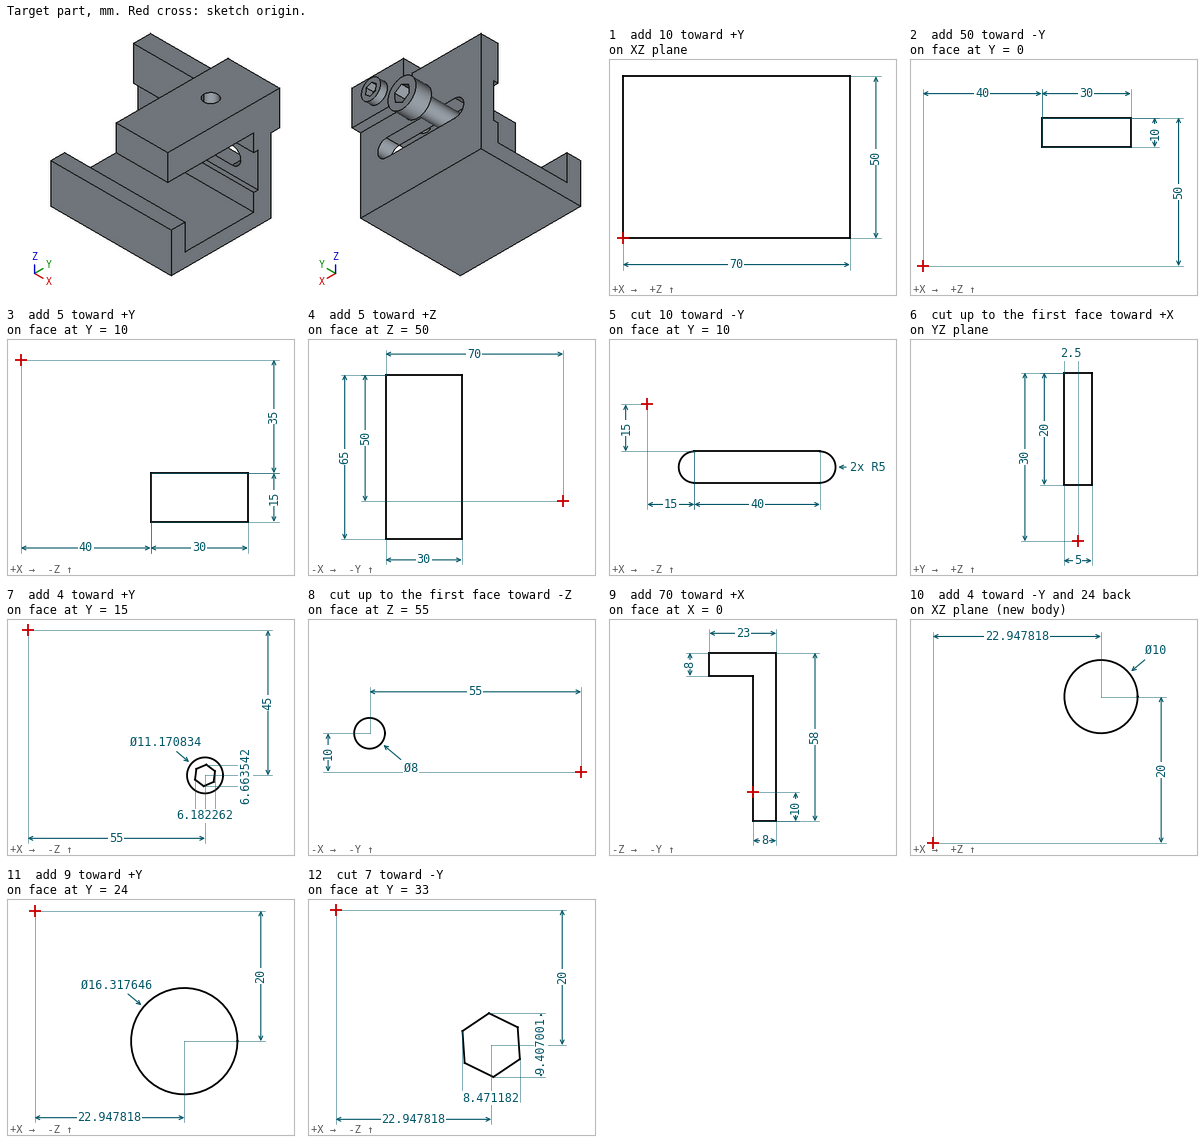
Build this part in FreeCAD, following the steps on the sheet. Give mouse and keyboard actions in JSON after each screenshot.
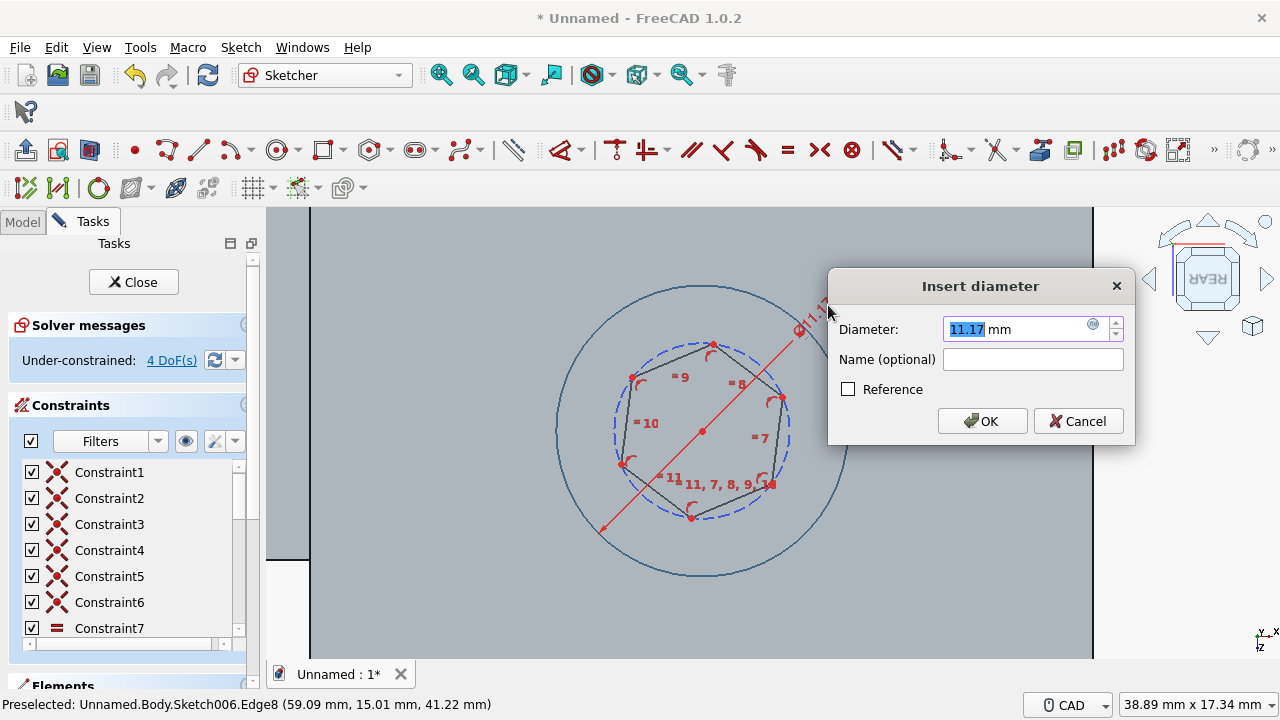
{"action": "type", "text": "11.170834"}
{"action": "key", "text": "Return"}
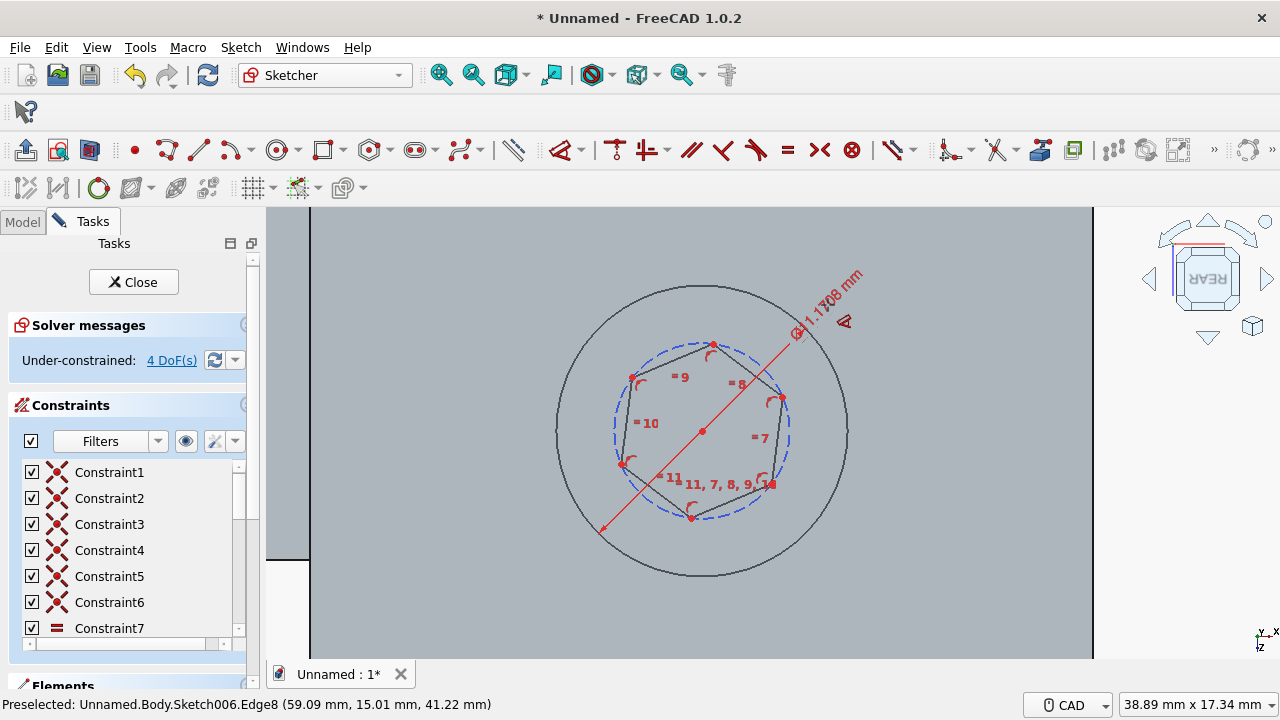
{"action": "left_click", "coordinate": [702, 431]}
{"action": "left_click", "coordinate": [498, 465]}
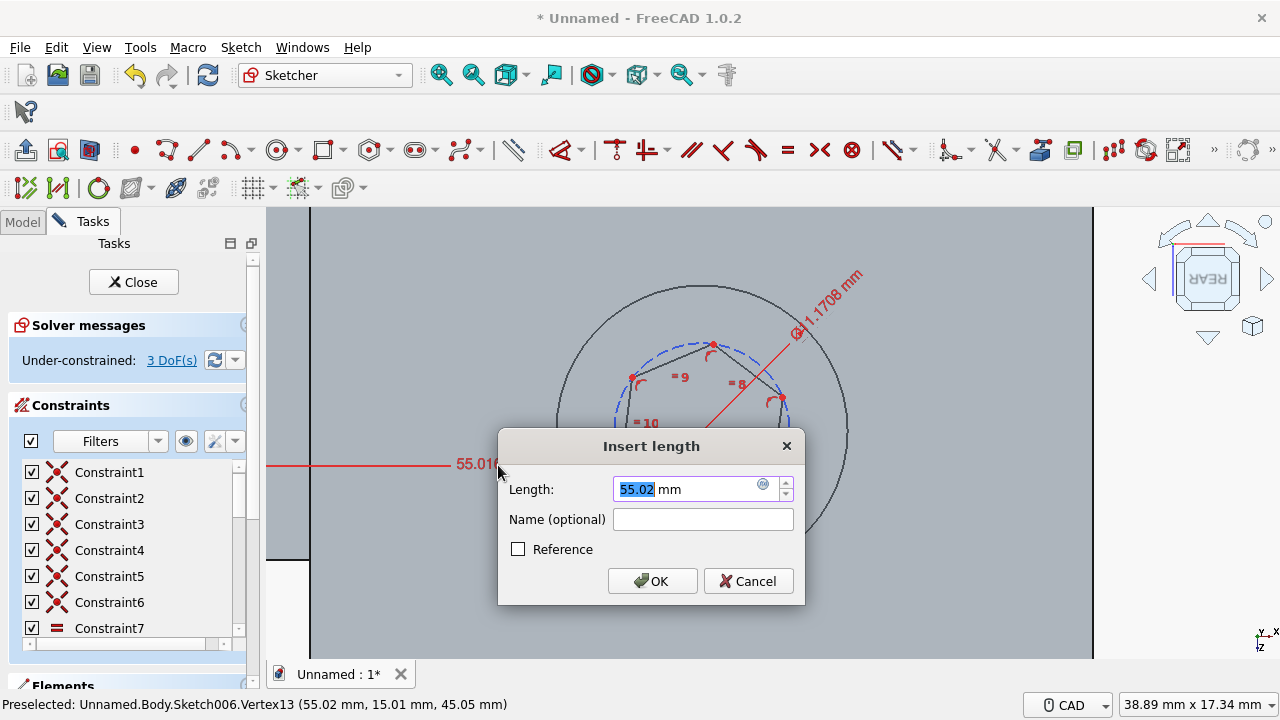
{"action": "type", "text": "55"}
{"action": "key", "text": "Return"}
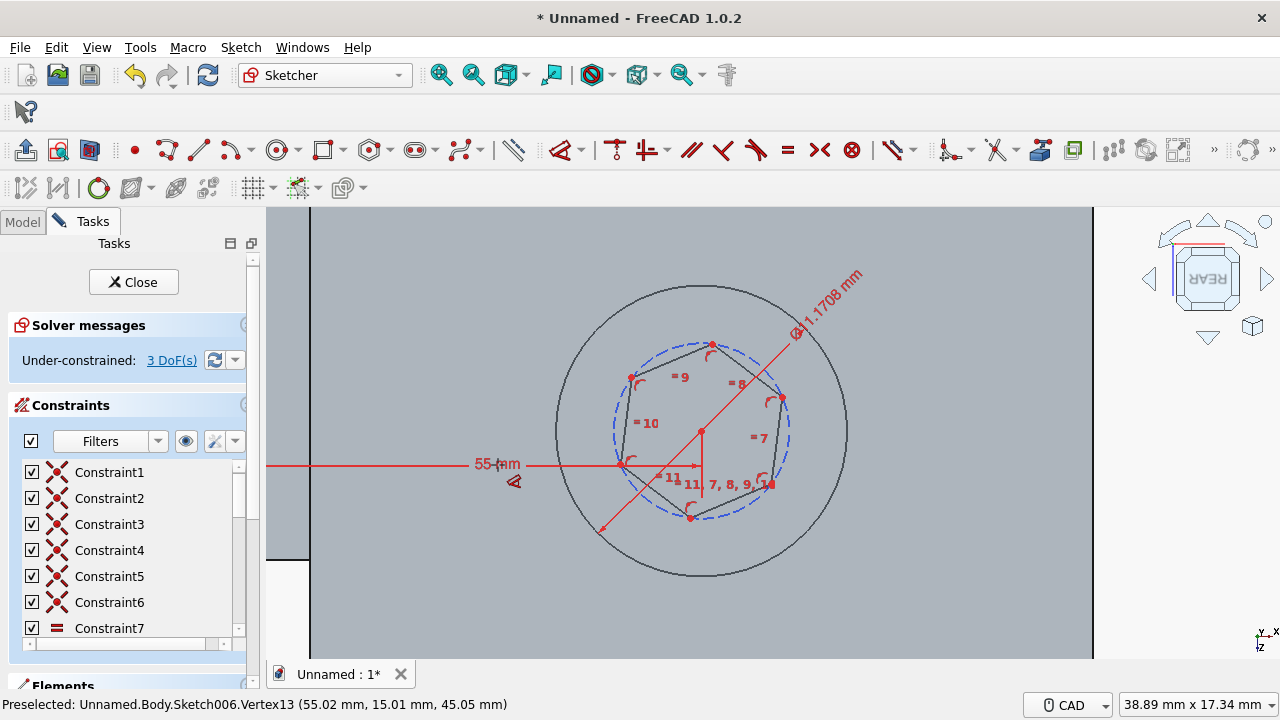
{"action": "left_click", "coordinate": [702, 431]}
{"action": "left_click", "coordinate": [736, 333]}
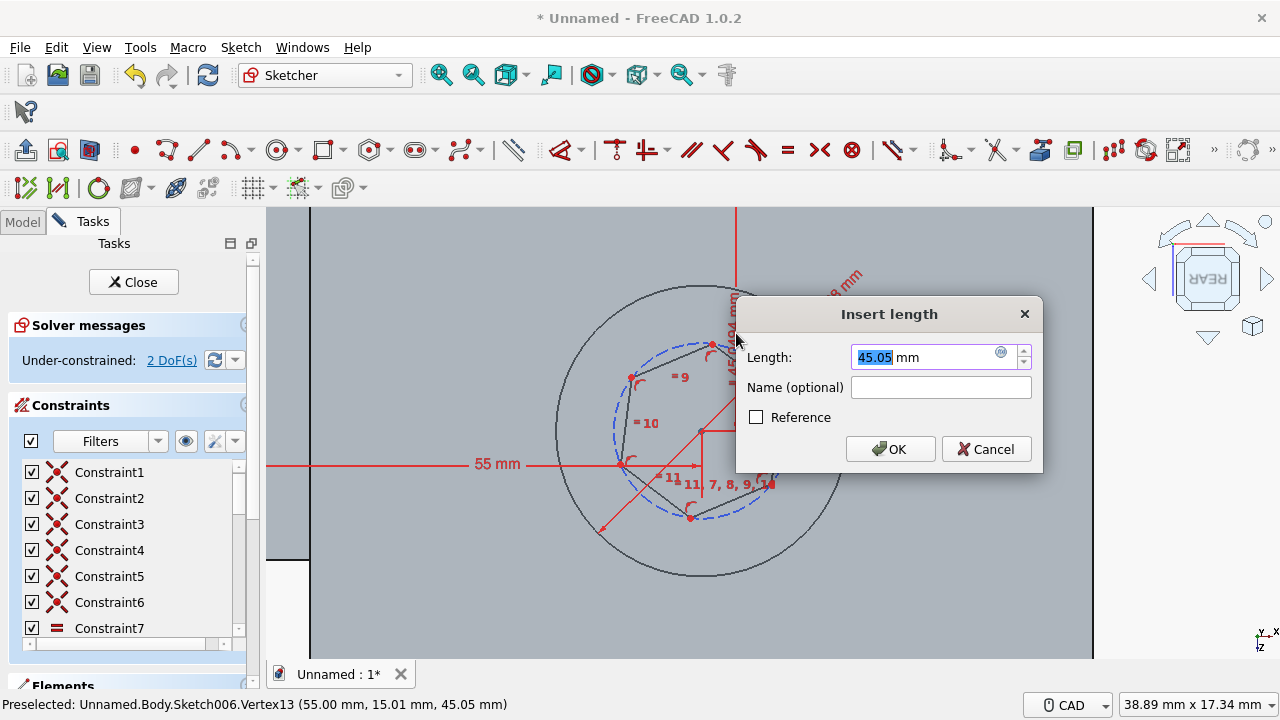
{"action": "type", "text": "45"}
{"action": "key", "text": "Return"}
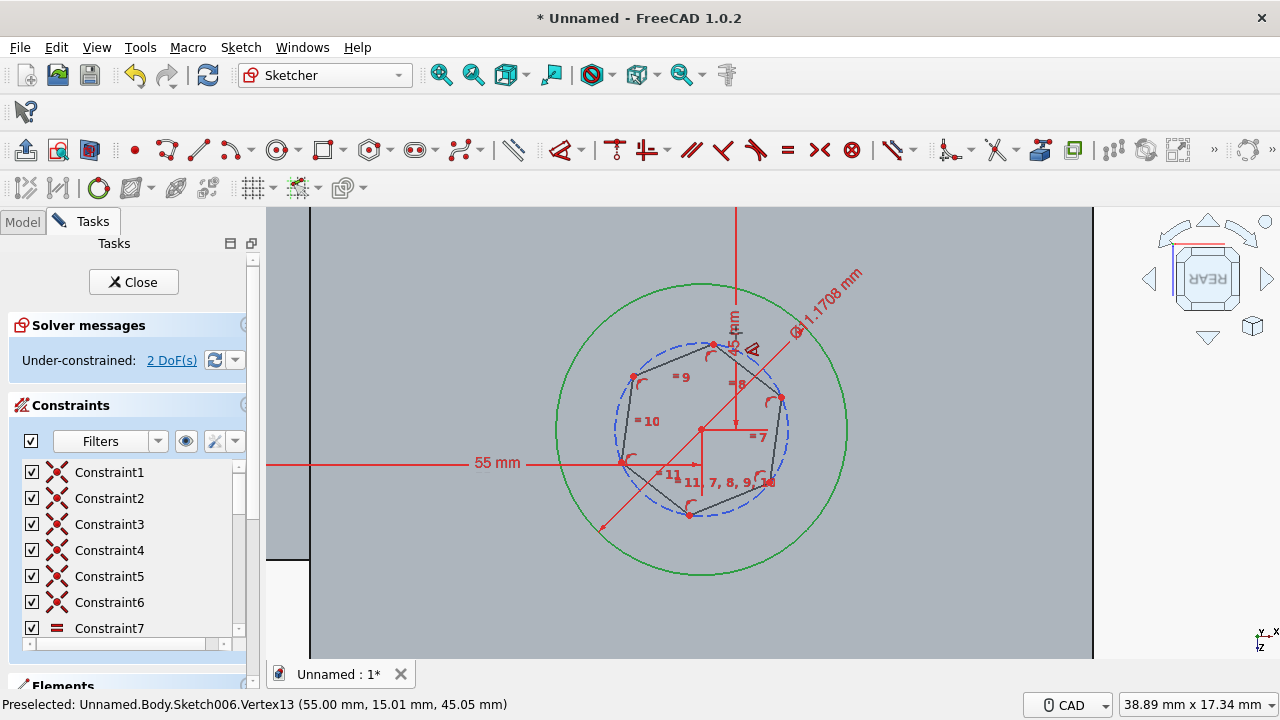
{"action": "left_click", "coordinate": [621, 462]}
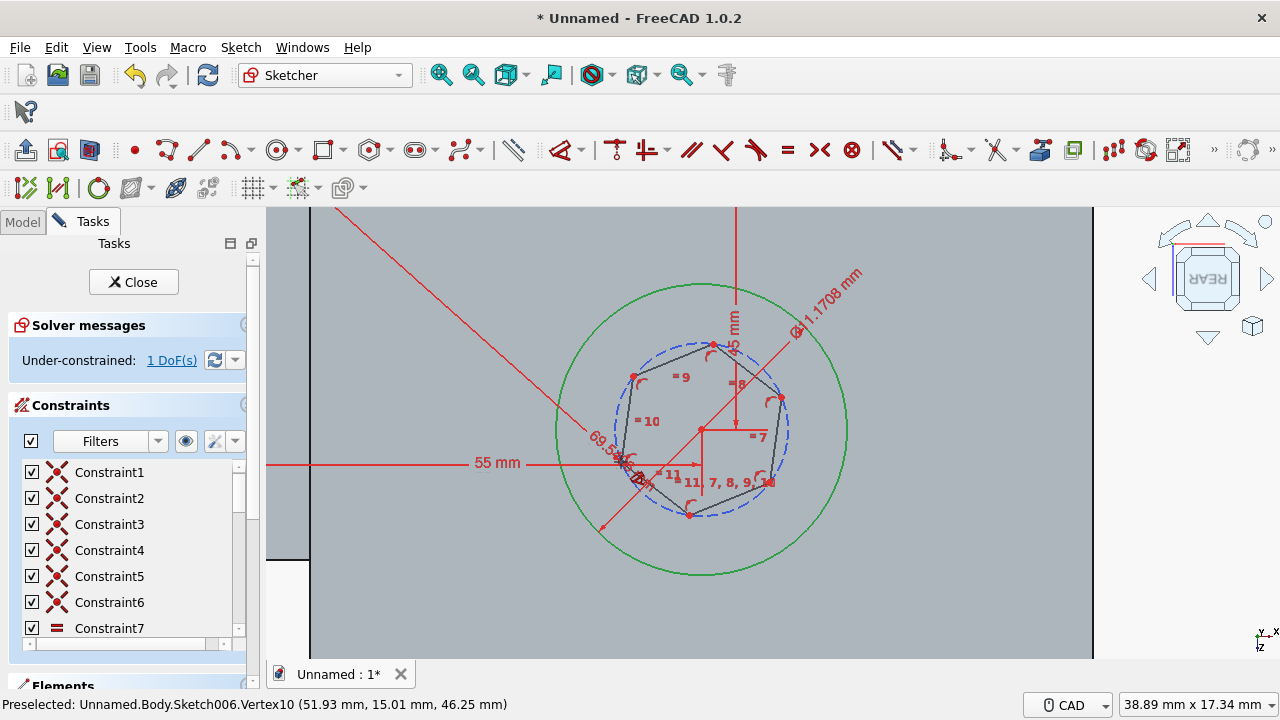
{"action": "left_click", "coordinate": [782, 397]}
{"action": "left_click", "coordinate": [702, 496]}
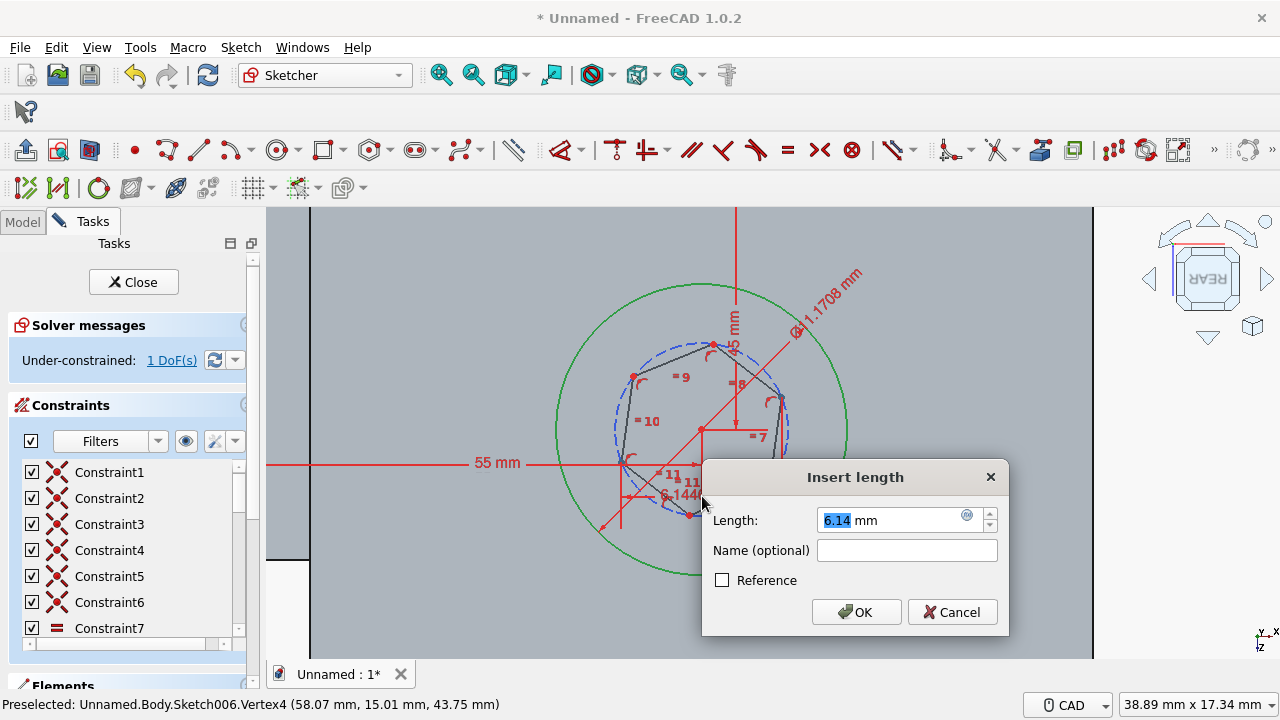
{"action": "type", "text": "6.182262"}
{"action": "key", "text": "Return"}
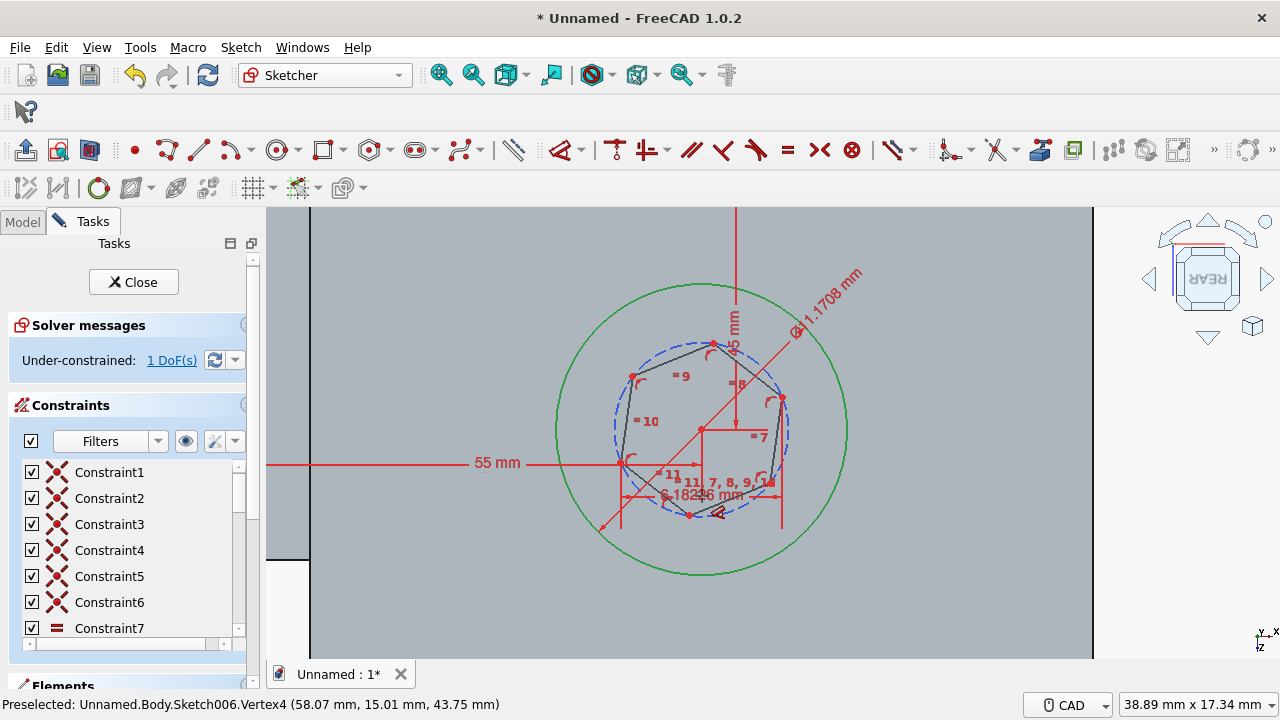
{"action": "left_click", "coordinate": [690, 516]}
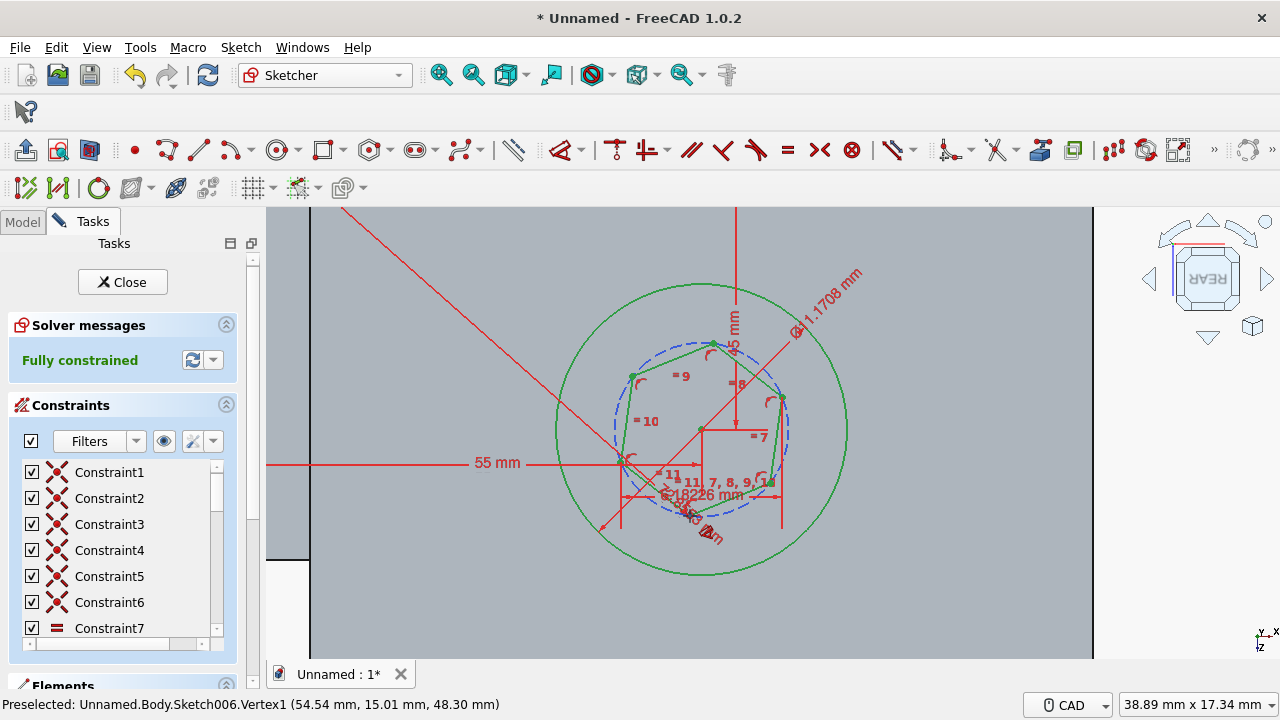
{"action": "left_click", "coordinate": [714, 344]}
{"action": "left_click", "coordinate": [656, 430]}